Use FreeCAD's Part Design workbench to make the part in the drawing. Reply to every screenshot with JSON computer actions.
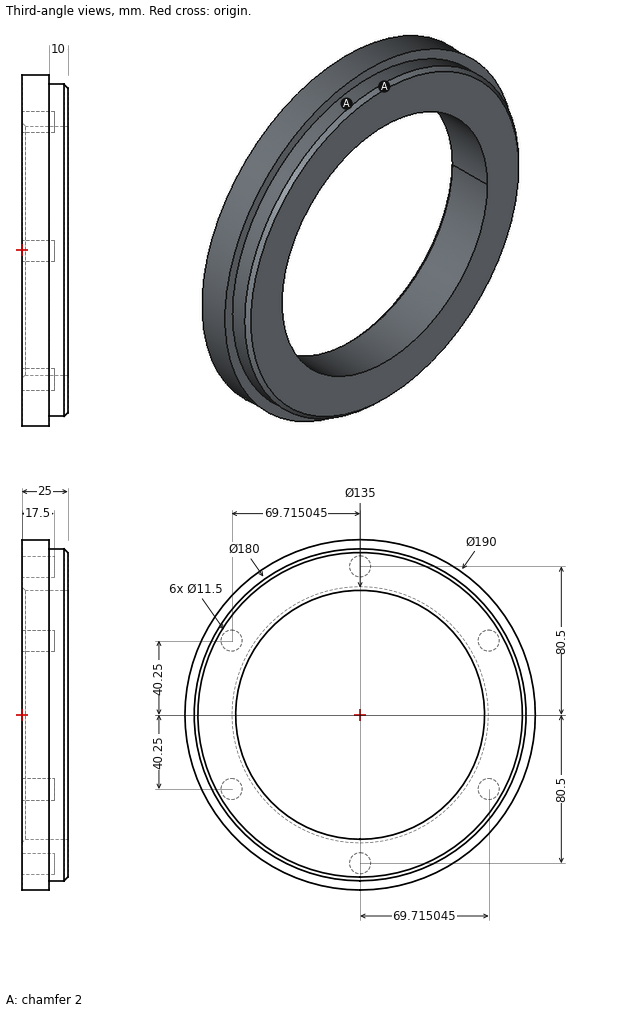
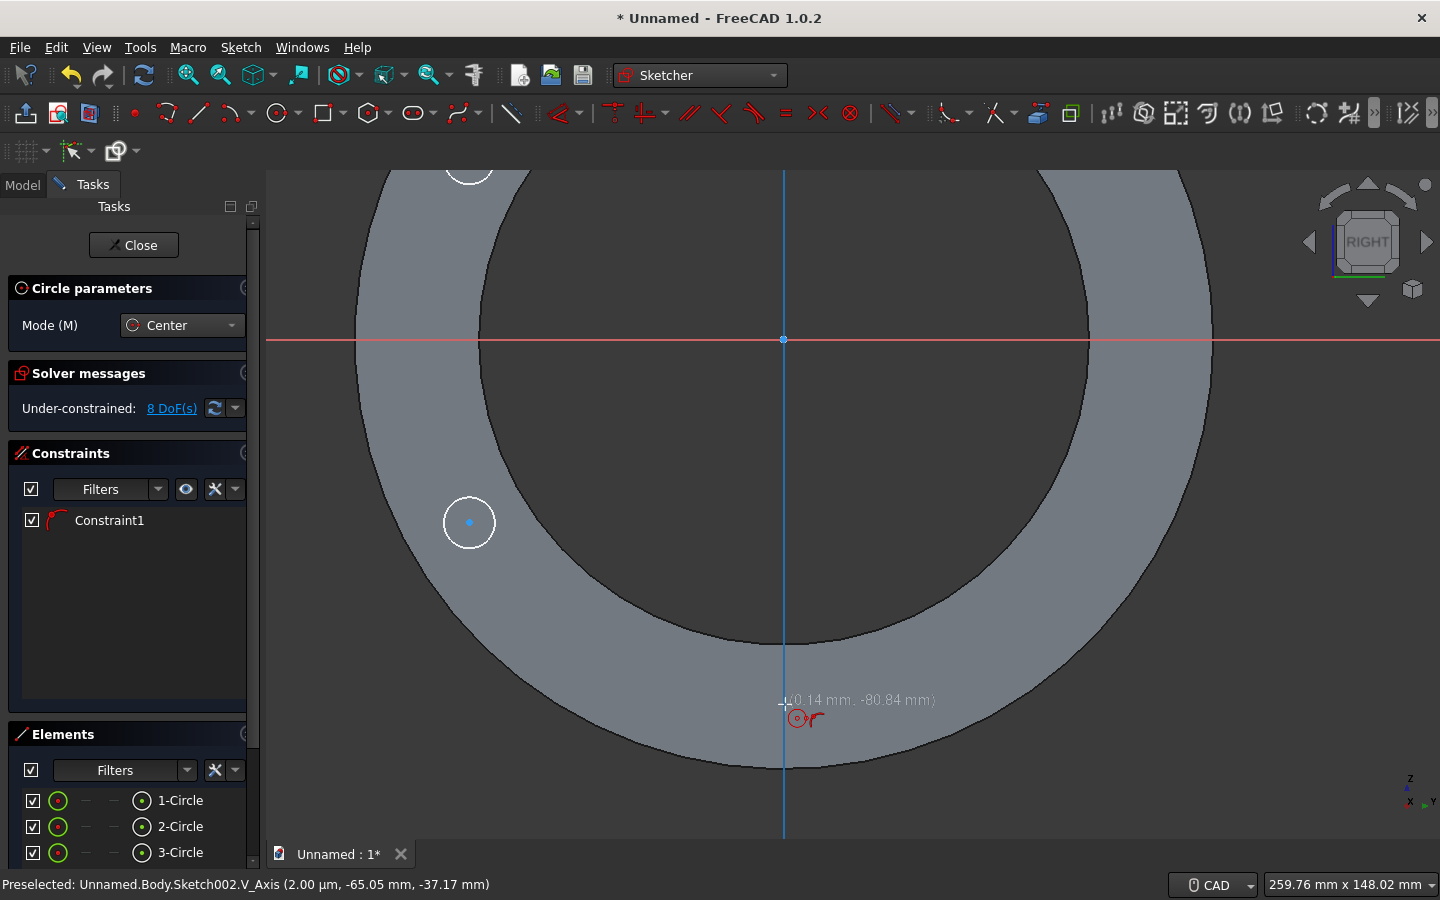
{"action": "left_click", "coordinate": [784, 704]}
{"action": "left_click", "coordinate": [802, 685]}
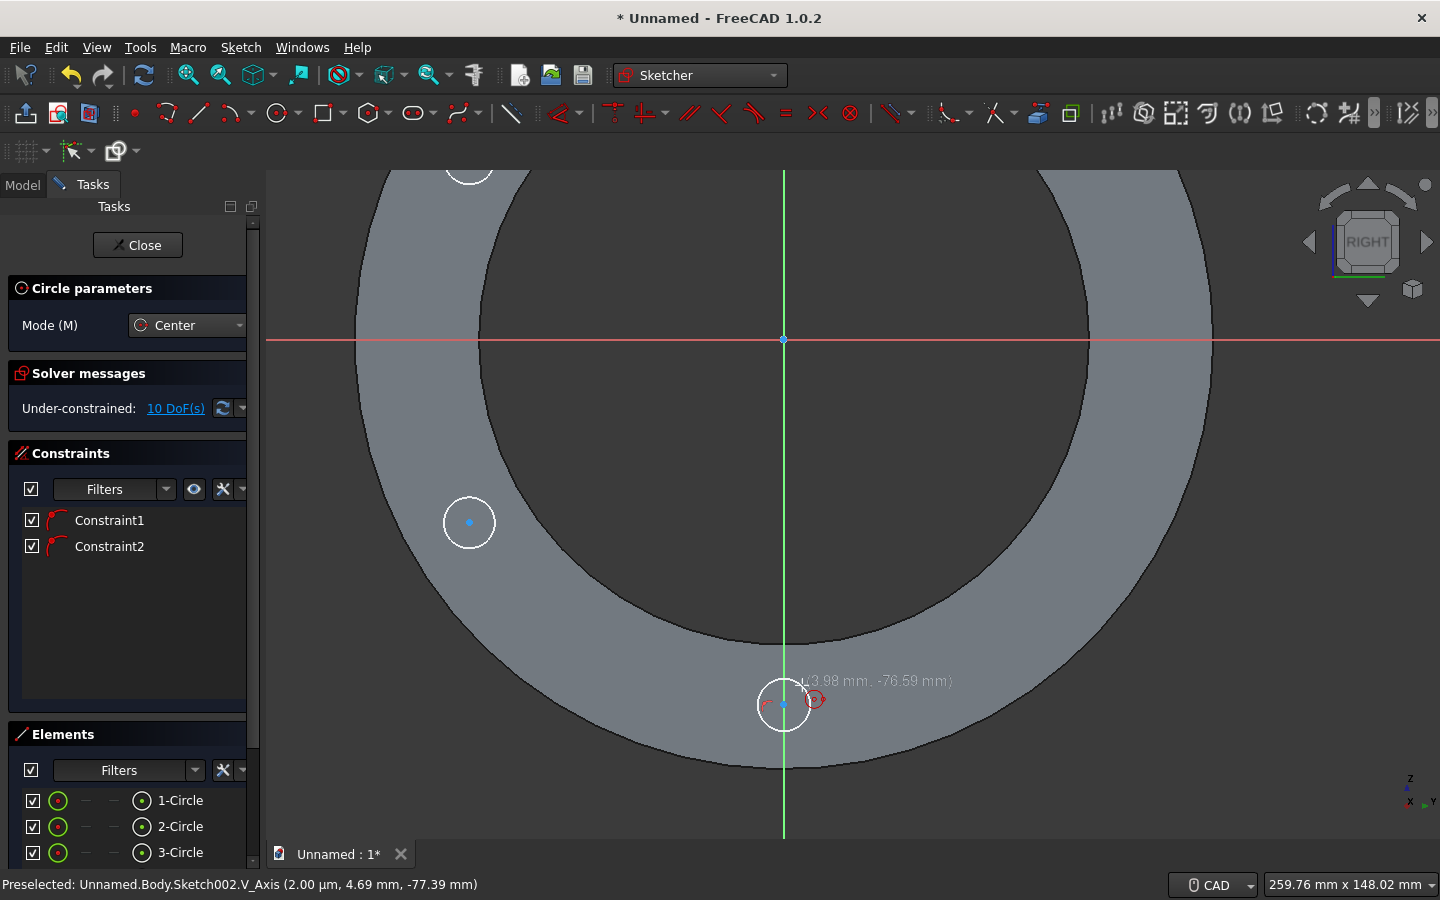
{"action": "left_click", "coordinate": [1099, 522]}
{"action": "left_click", "coordinate": [1117, 503]}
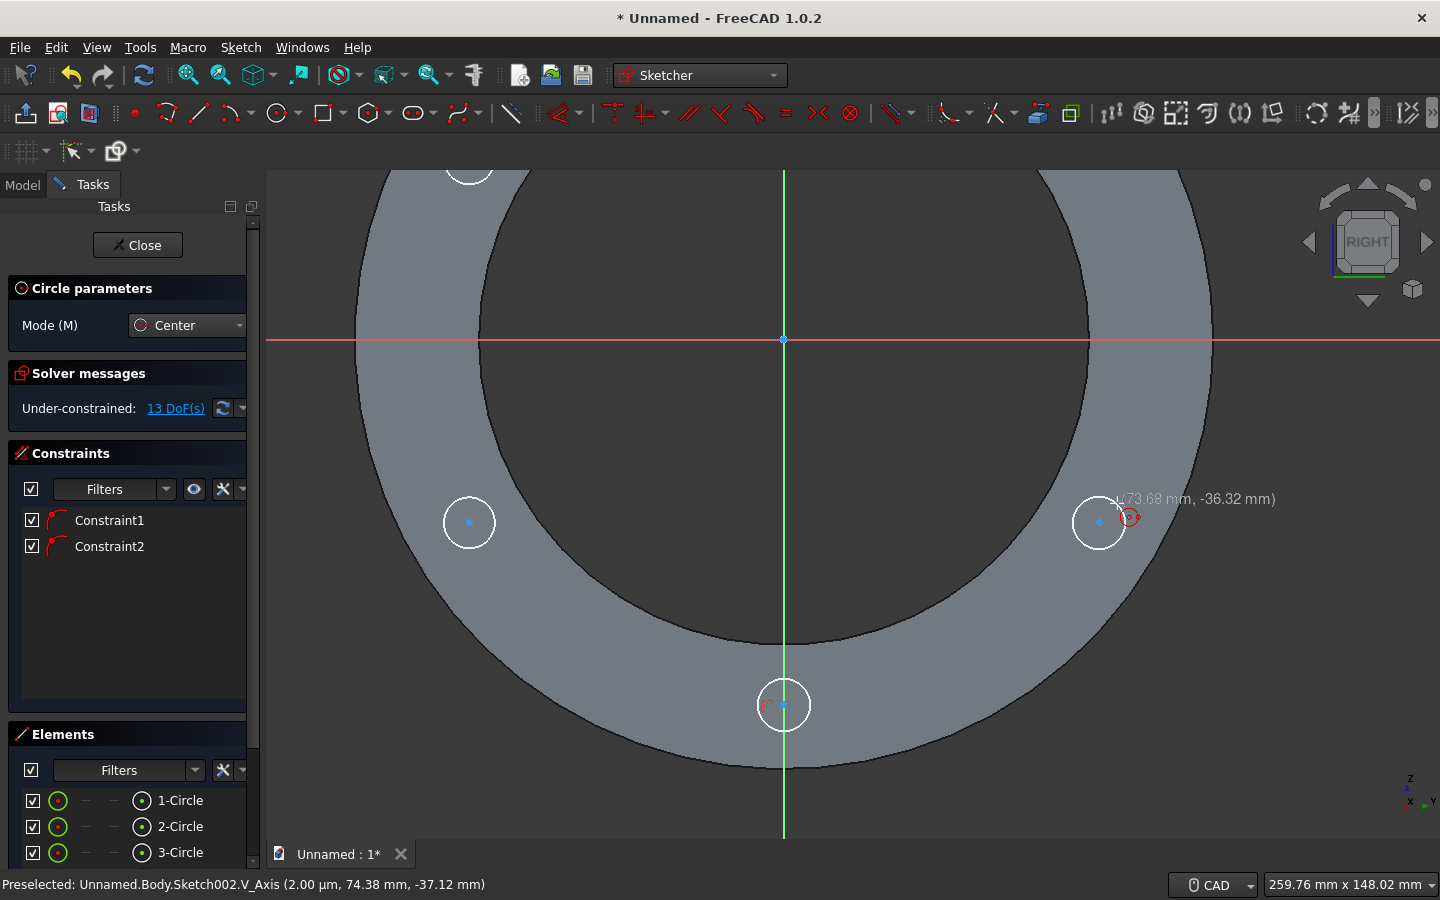
{"action": "scroll", "coordinate": [785, 705], "scroll_direction": "down", "scroll_amount": 3}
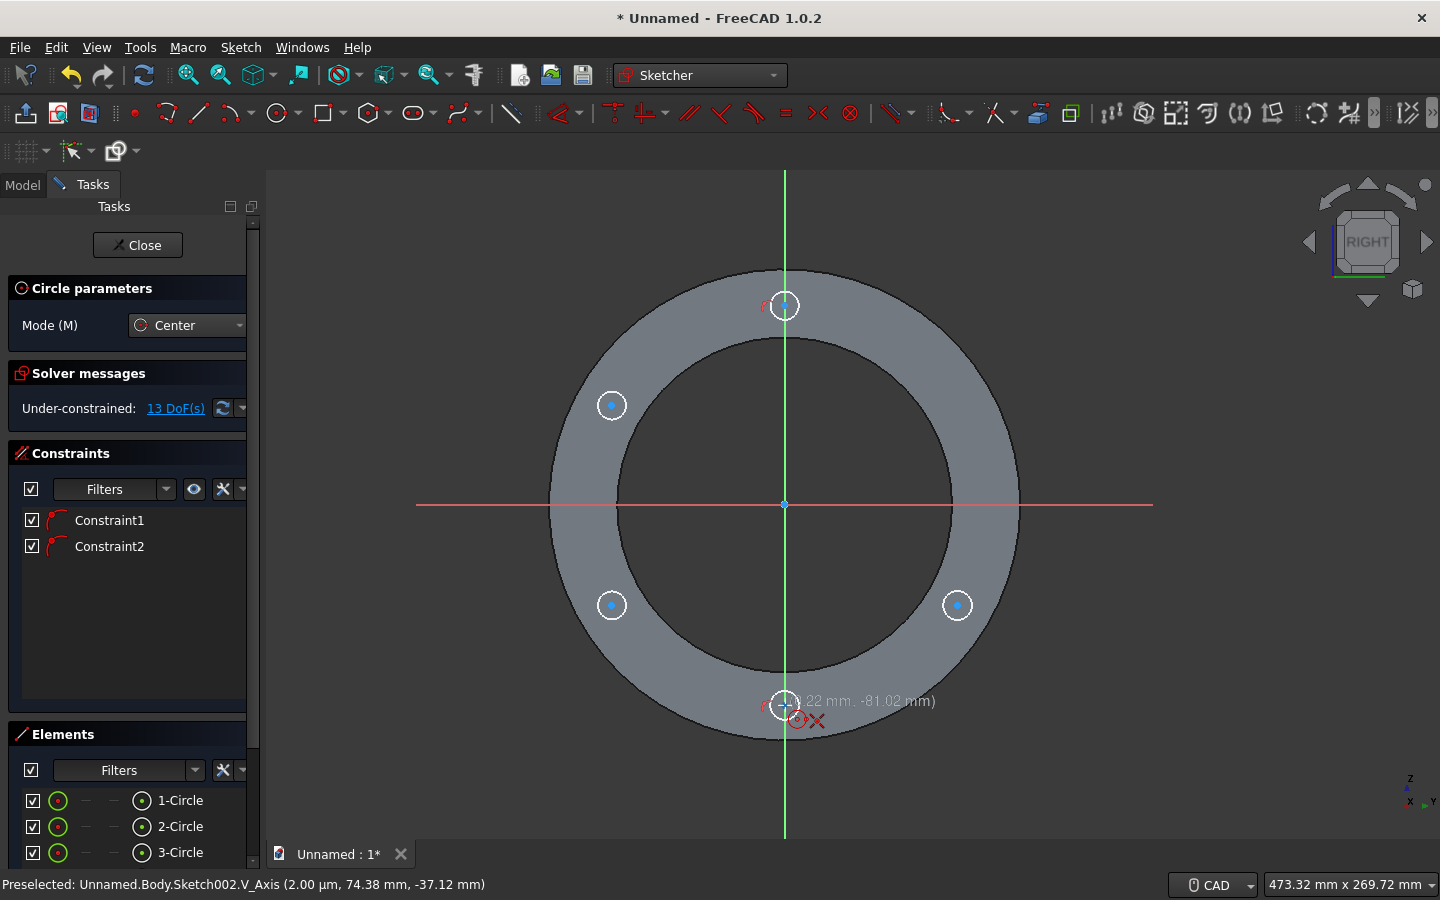
{"action": "scroll", "coordinate": [958, 405], "scroll_direction": "up", "scroll_amount": 3}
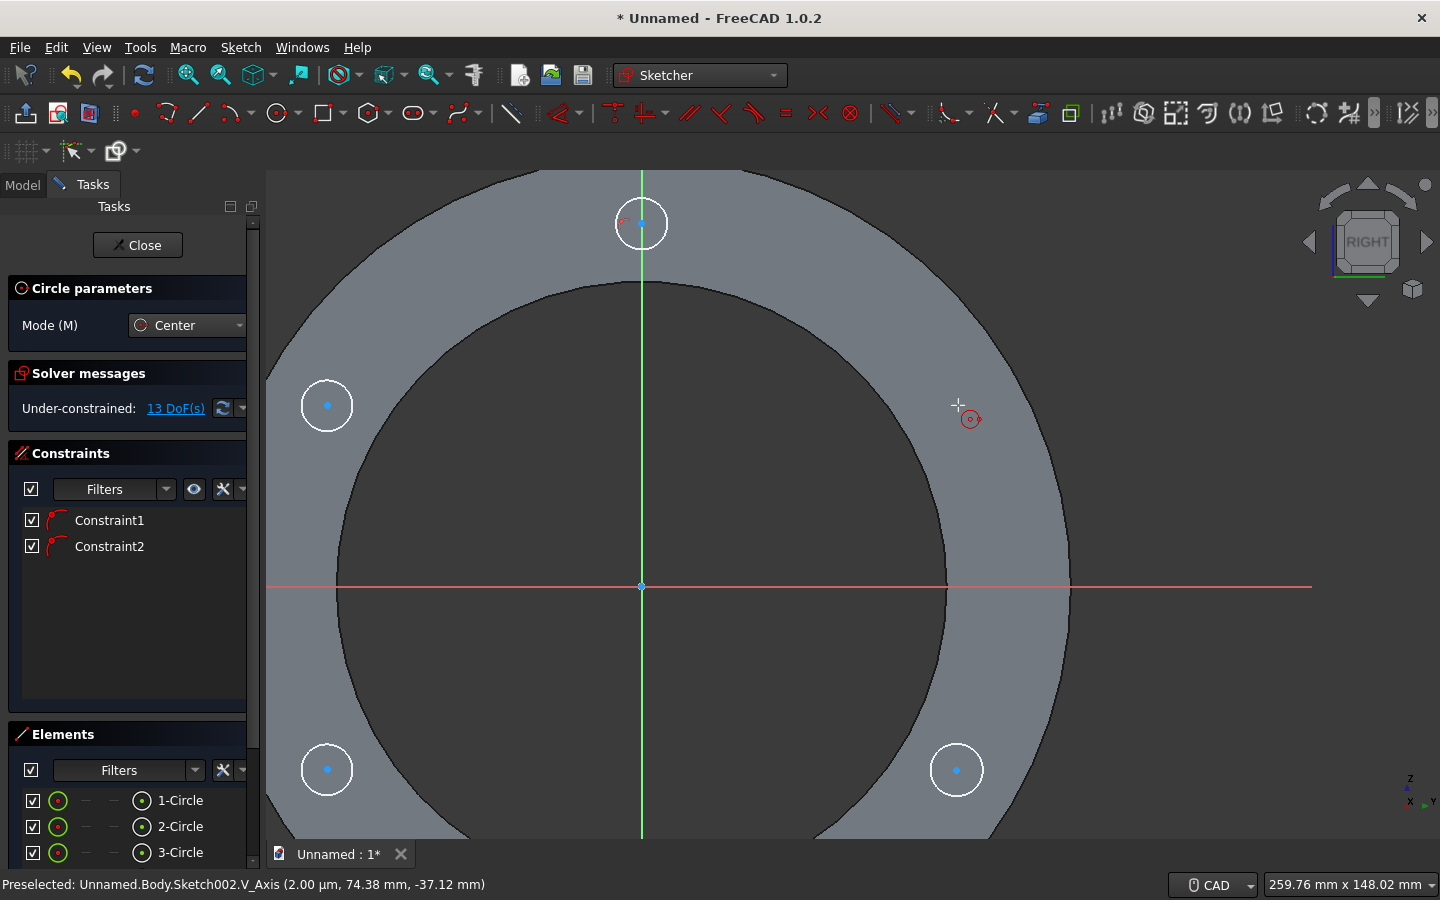
{"action": "left_click", "coordinate": [957, 405]}
{"action": "left_click", "coordinate": [975, 387]}
{"action": "key", "text": "Escape"}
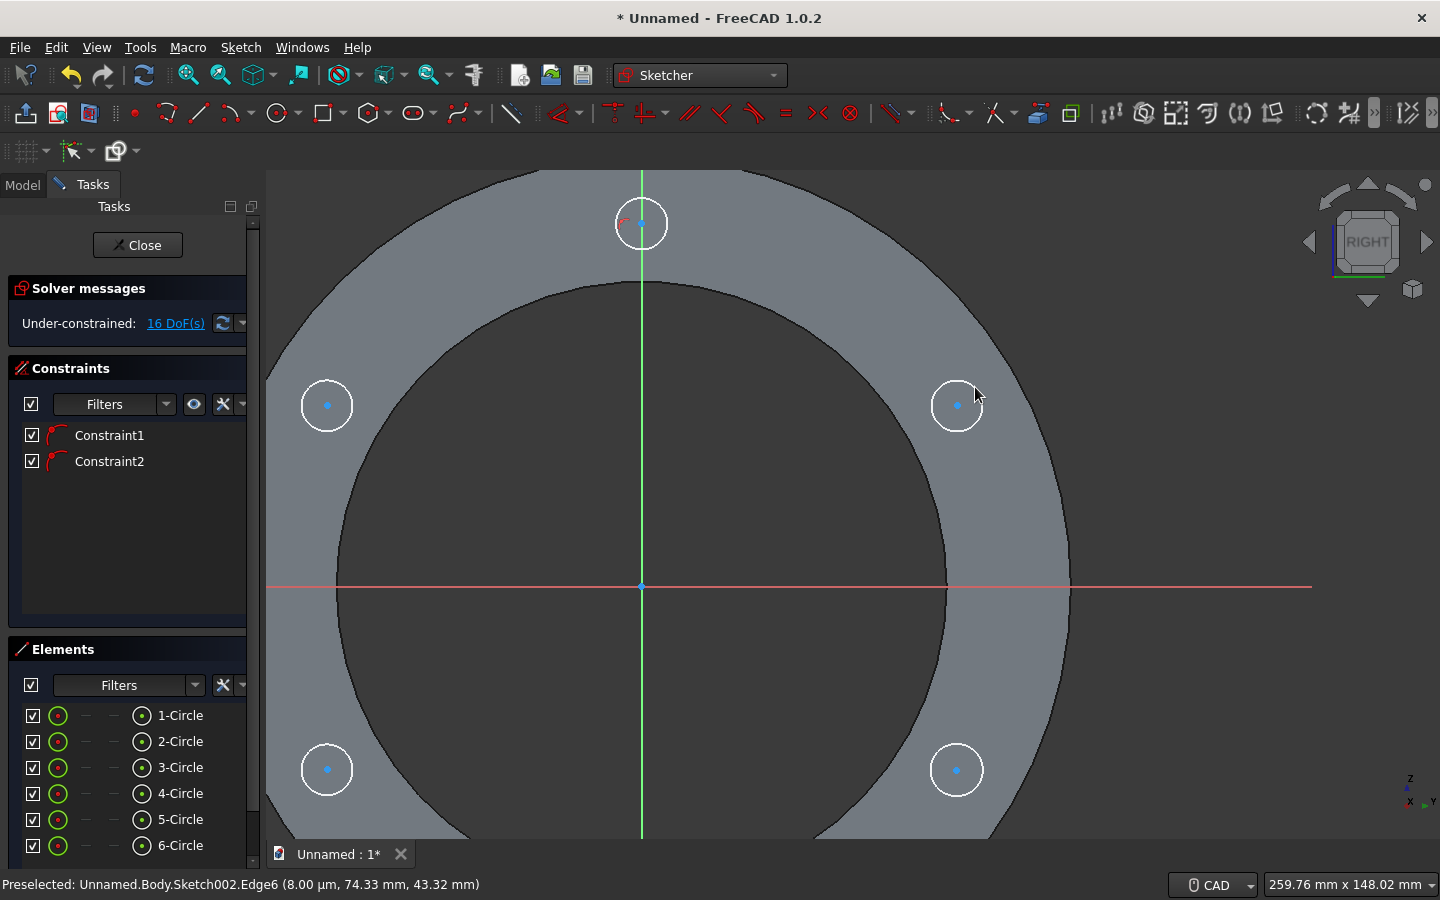
{"action": "left_click", "coordinate": [345, 388]}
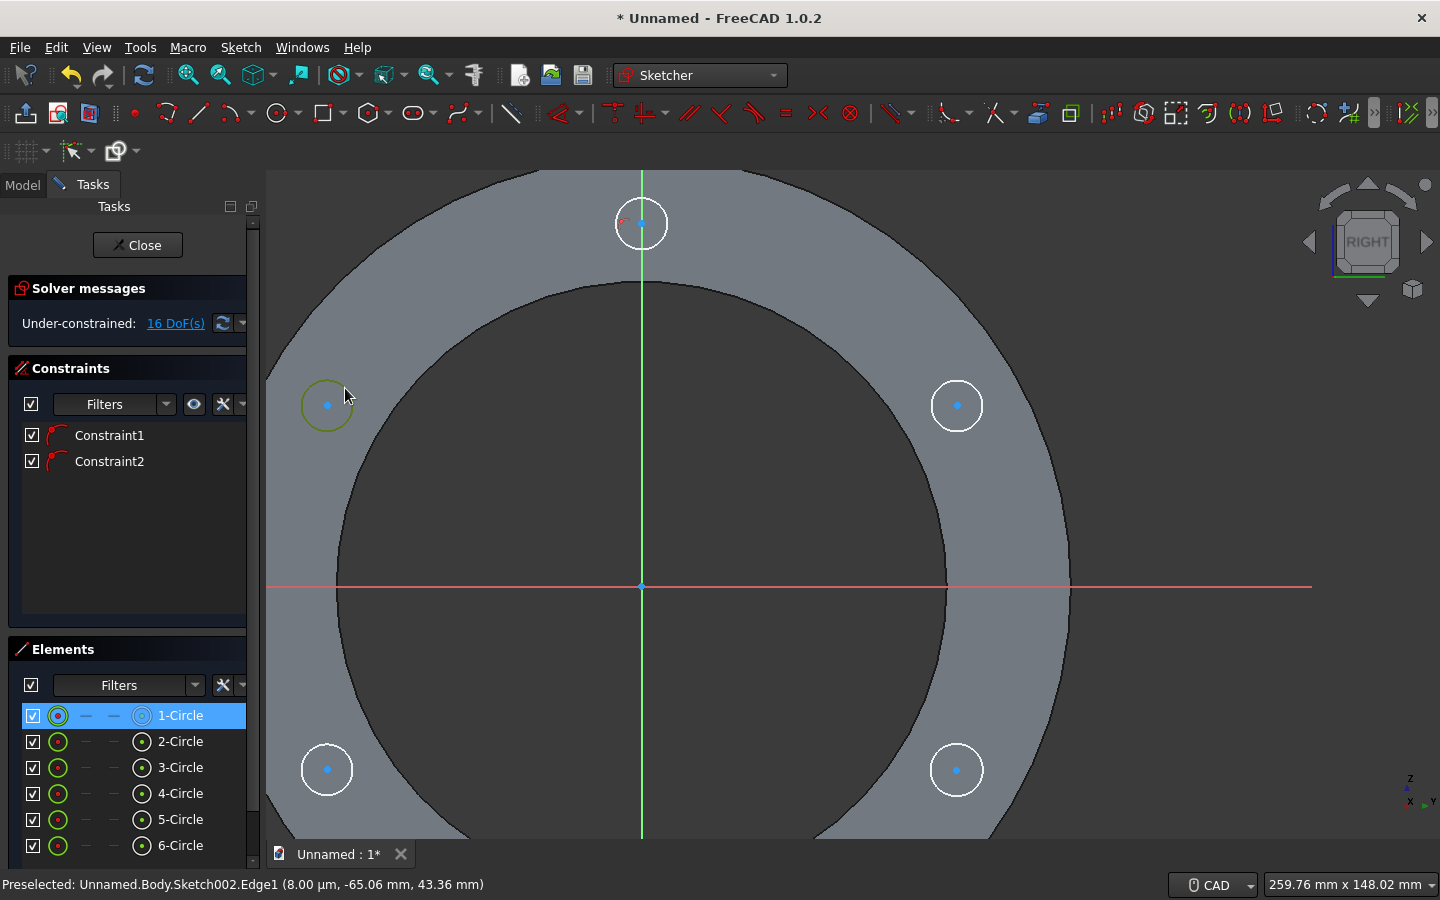
{"action": "left_click", "coordinate": [660, 206]}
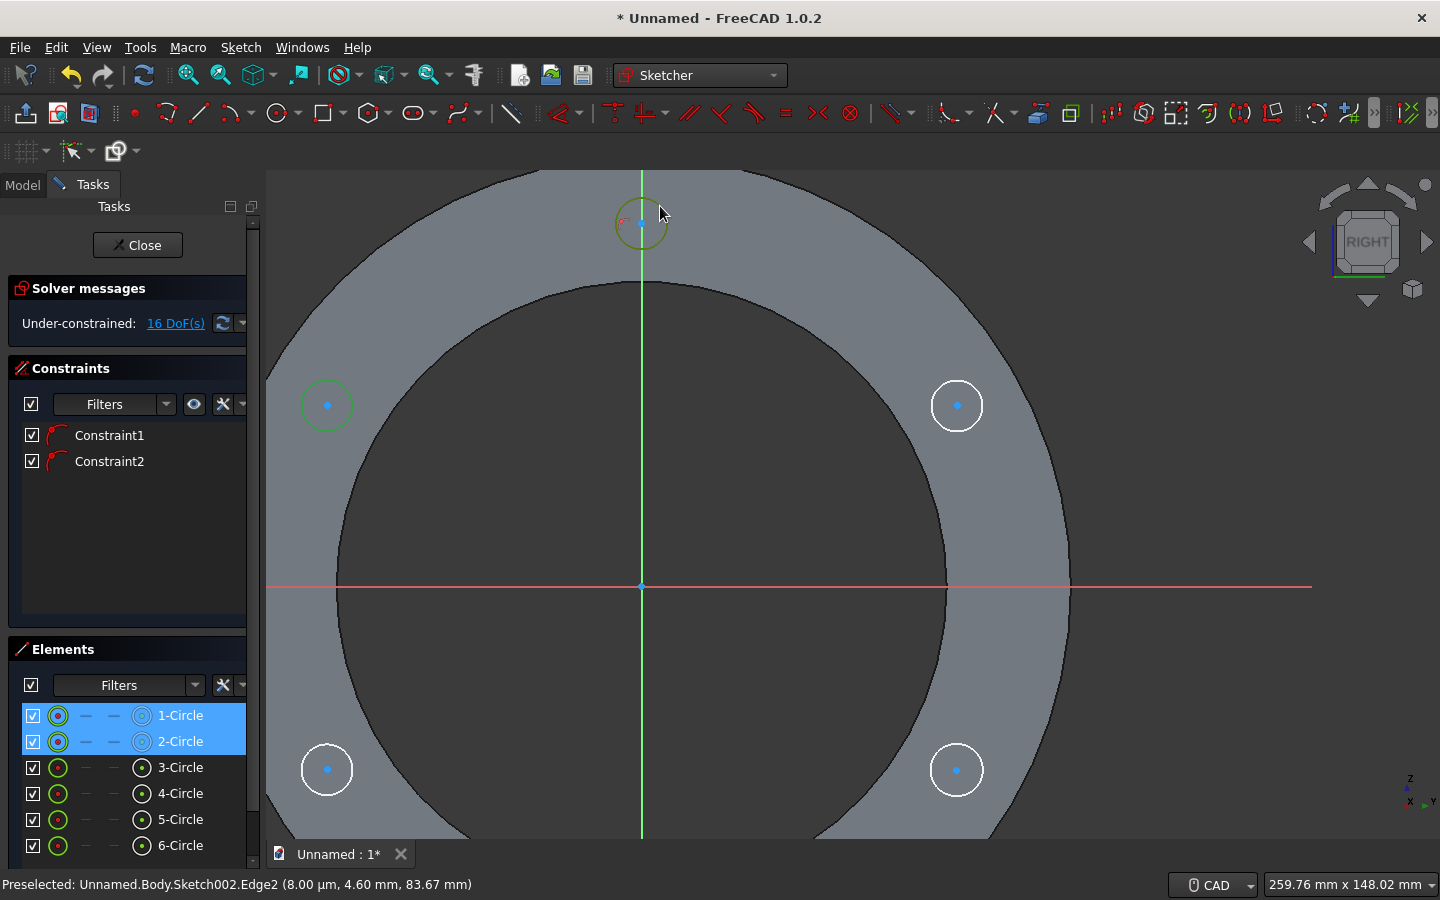
{"action": "left_click", "coordinate": [345, 752]}